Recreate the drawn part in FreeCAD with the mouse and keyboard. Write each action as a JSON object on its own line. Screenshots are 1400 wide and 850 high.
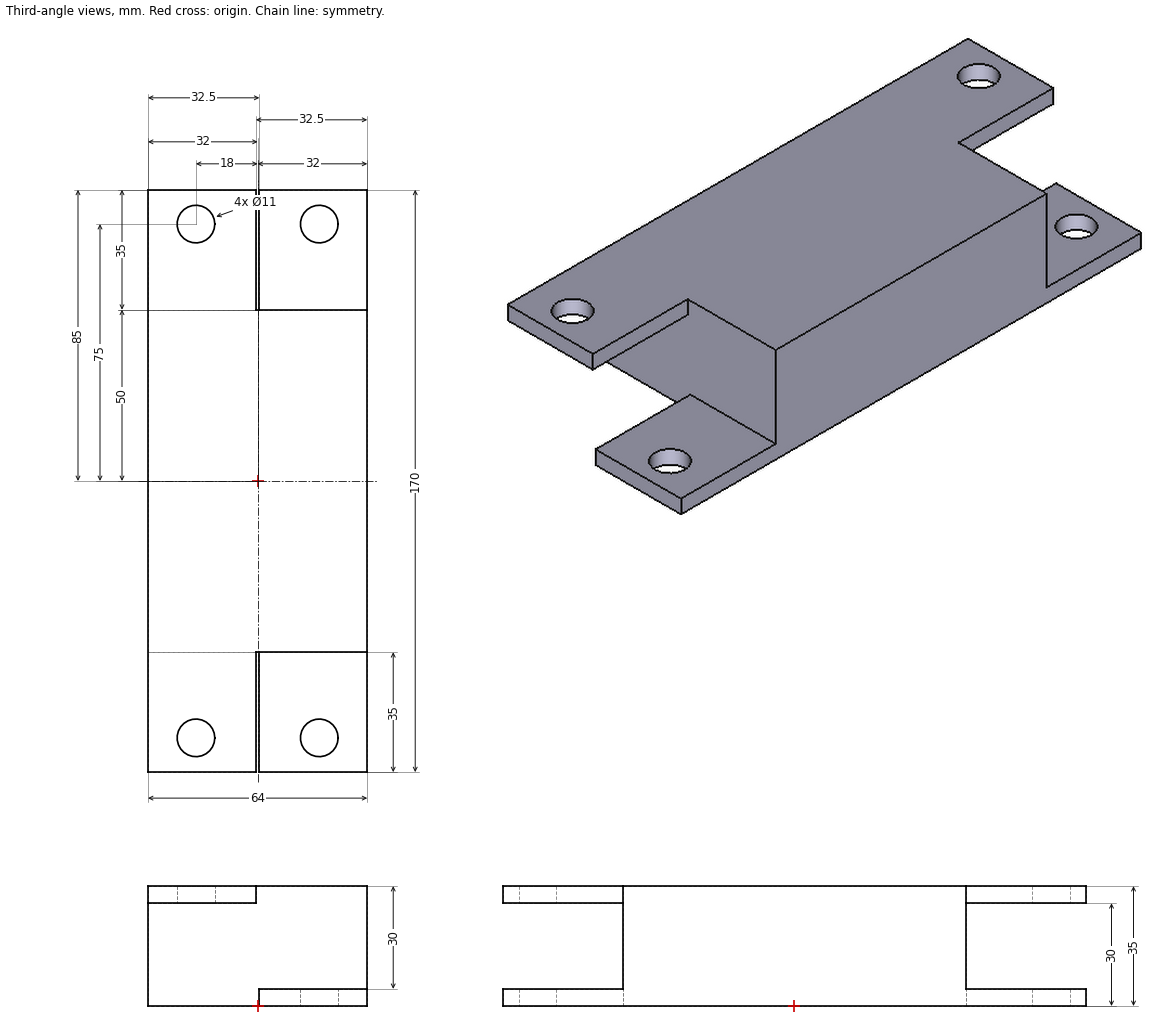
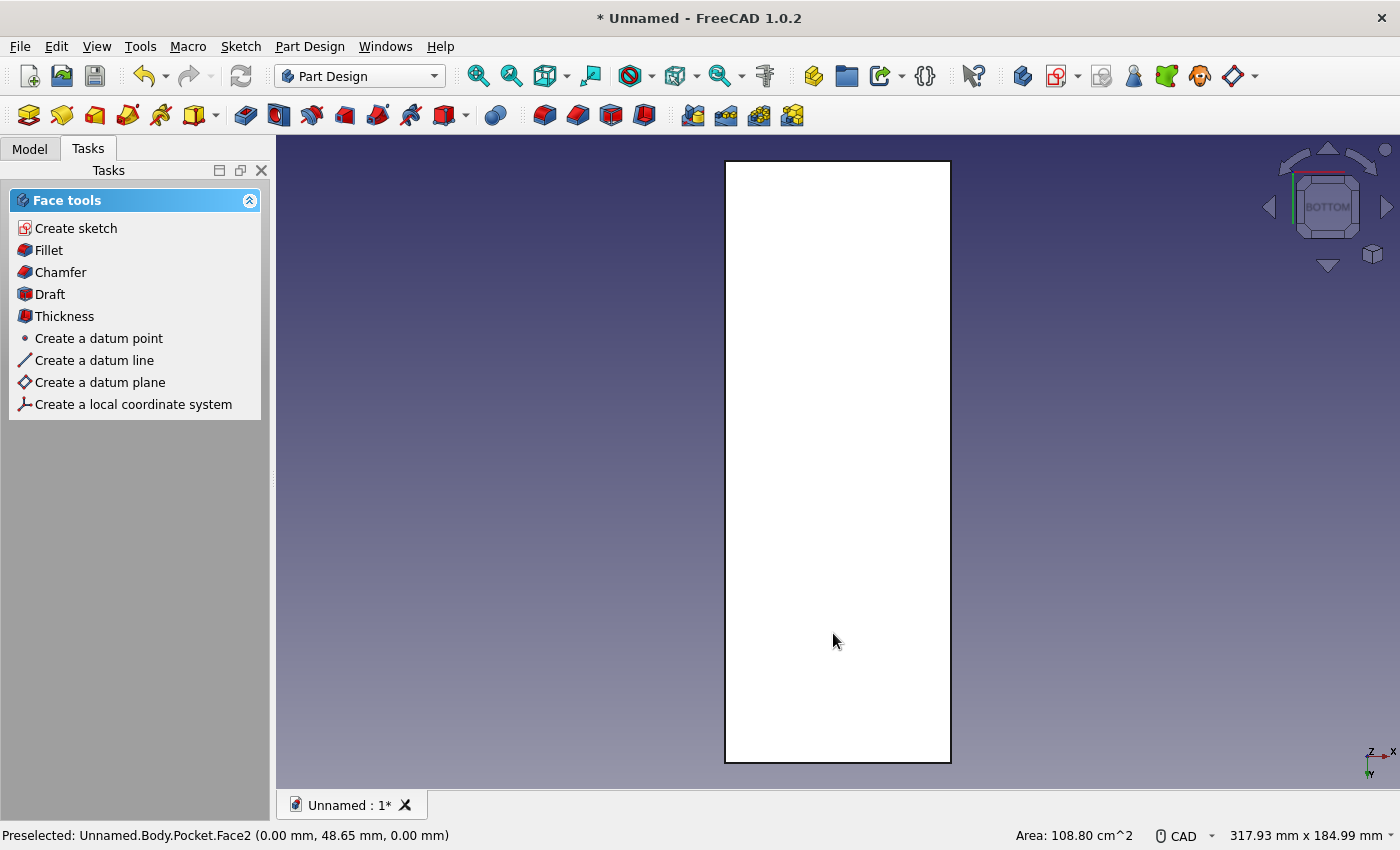
{"action": "left_click", "coordinate": [1056, 76]}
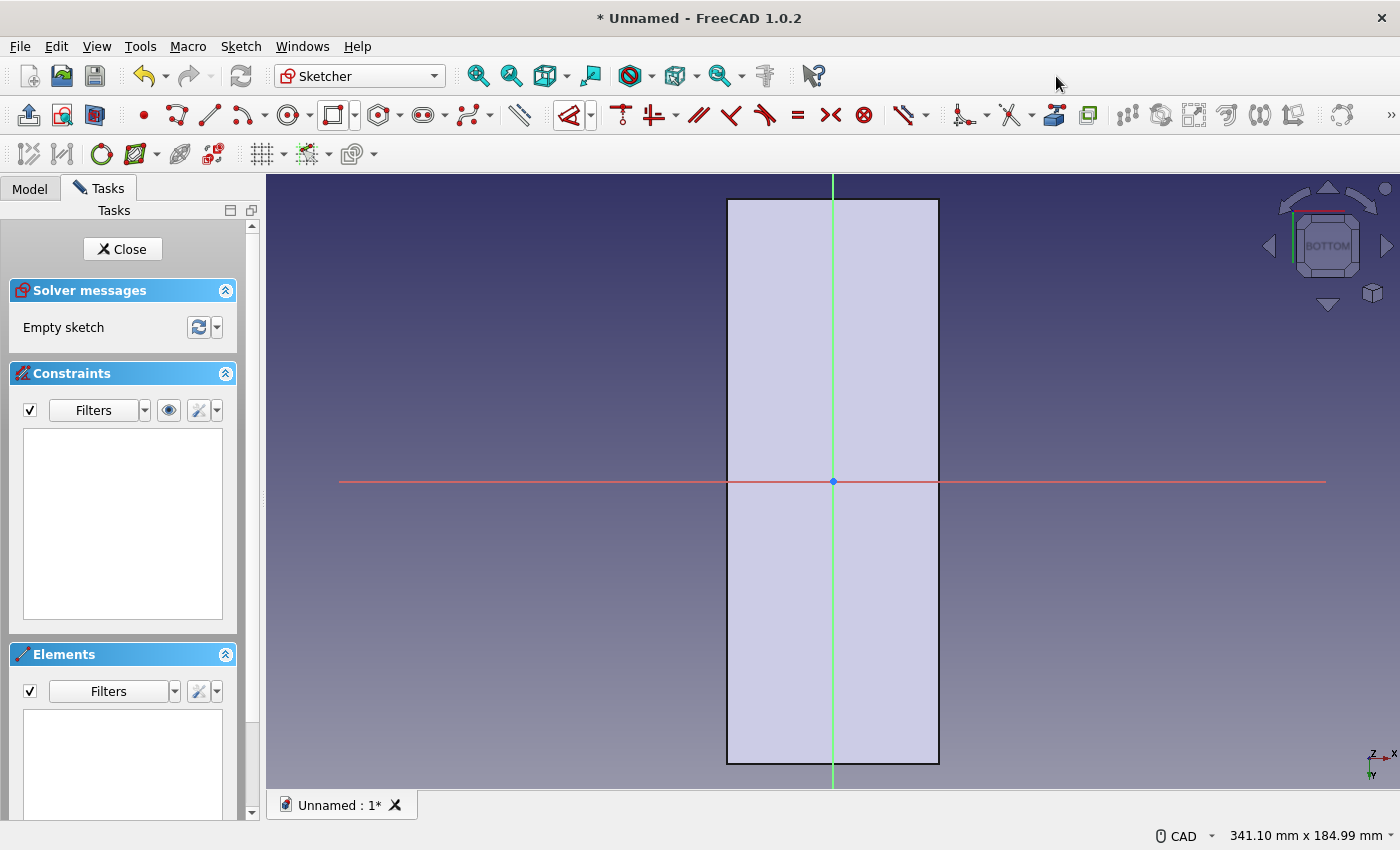
{"action": "scroll", "coordinate": [732, 481], "scroll_direction": "down", "scroll_amount": 2}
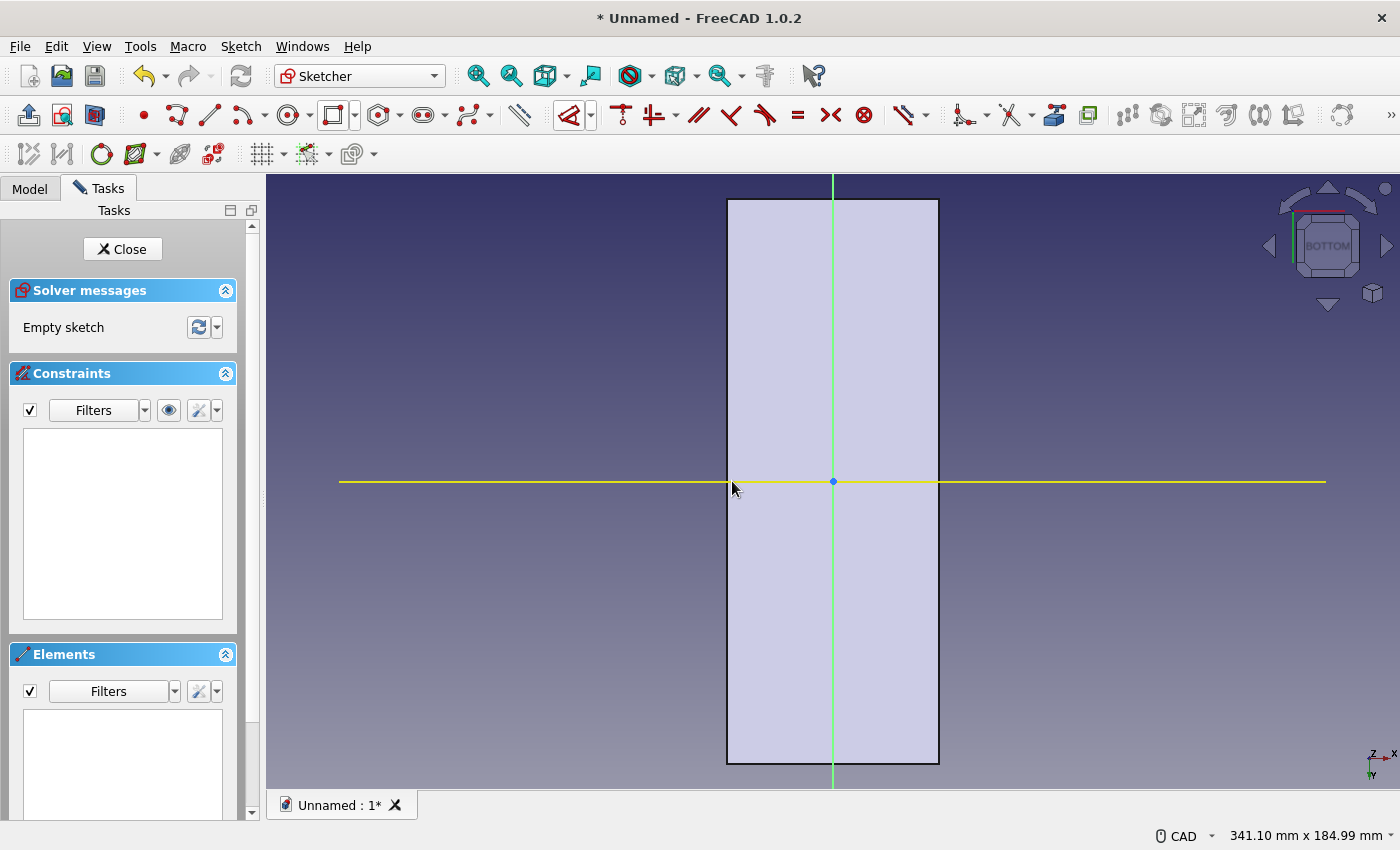
{"action": "left_click", "coordinate": [332, 116]}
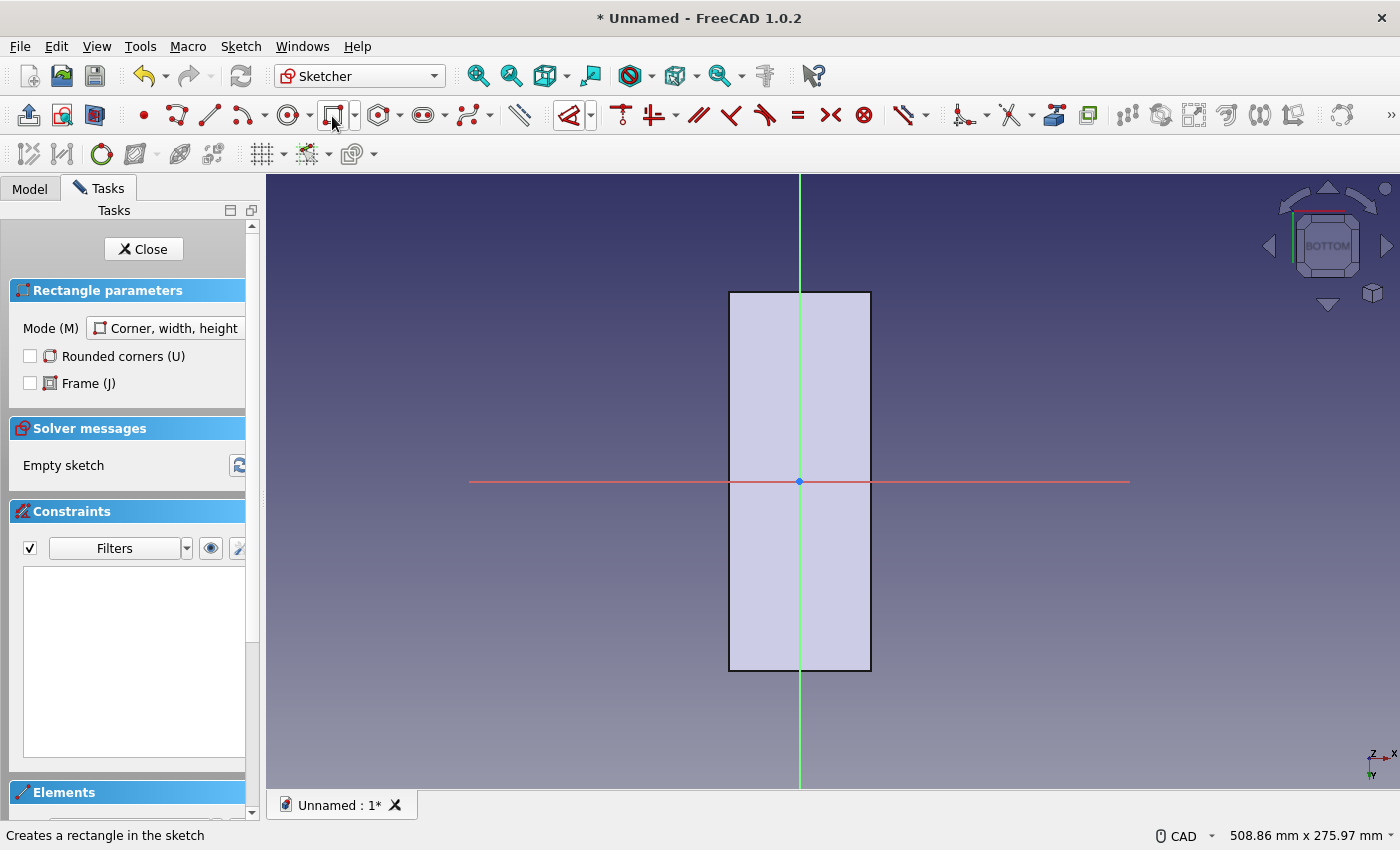
{"action": "left_click", "coordinate": [729, 593]}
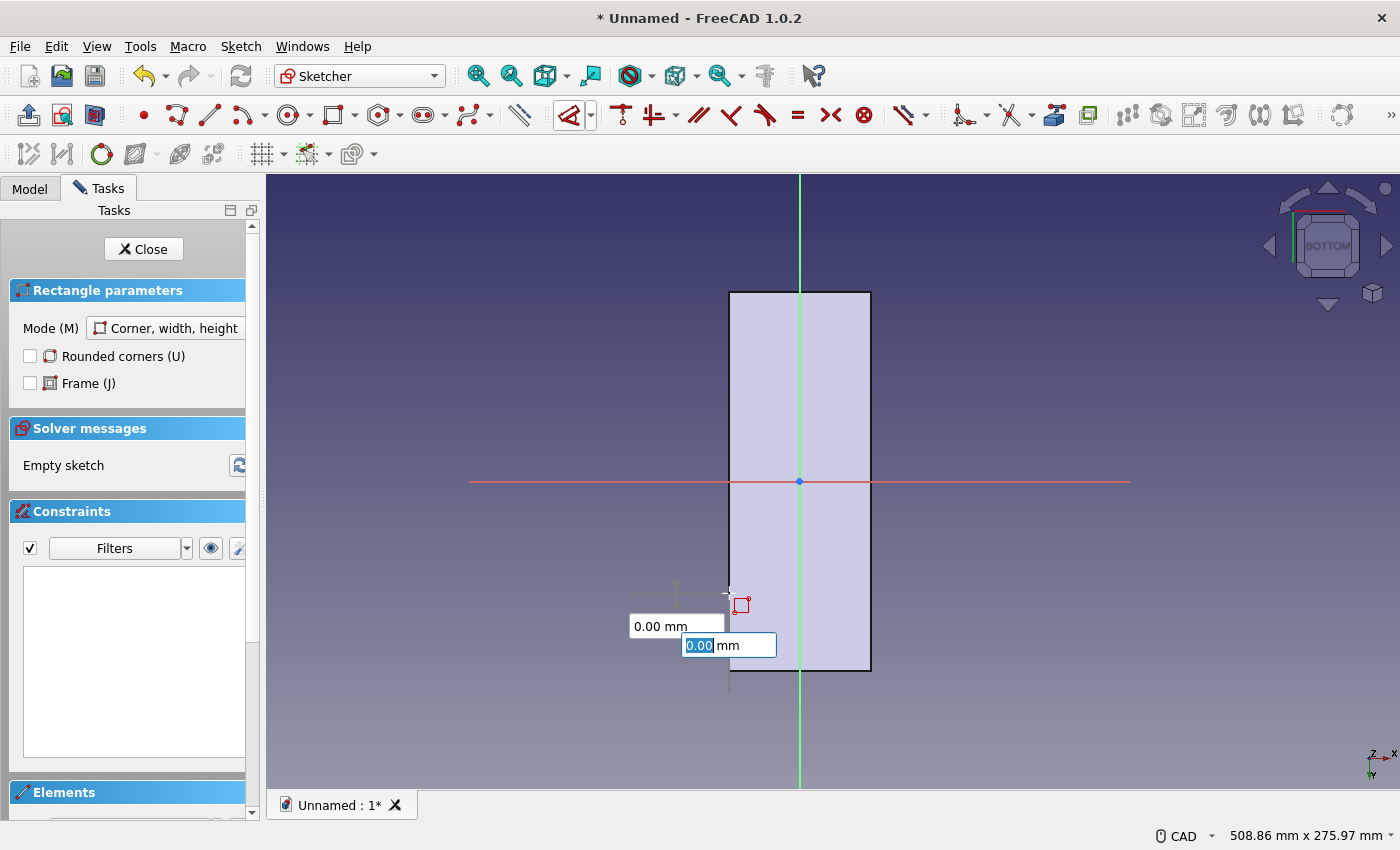
{"action": "scroll", "coordinate": [801, 671], "scroll_direction": "up", "scroll_amount": 14}
{"action": "mouse_move", "coordinate": [793, 657]}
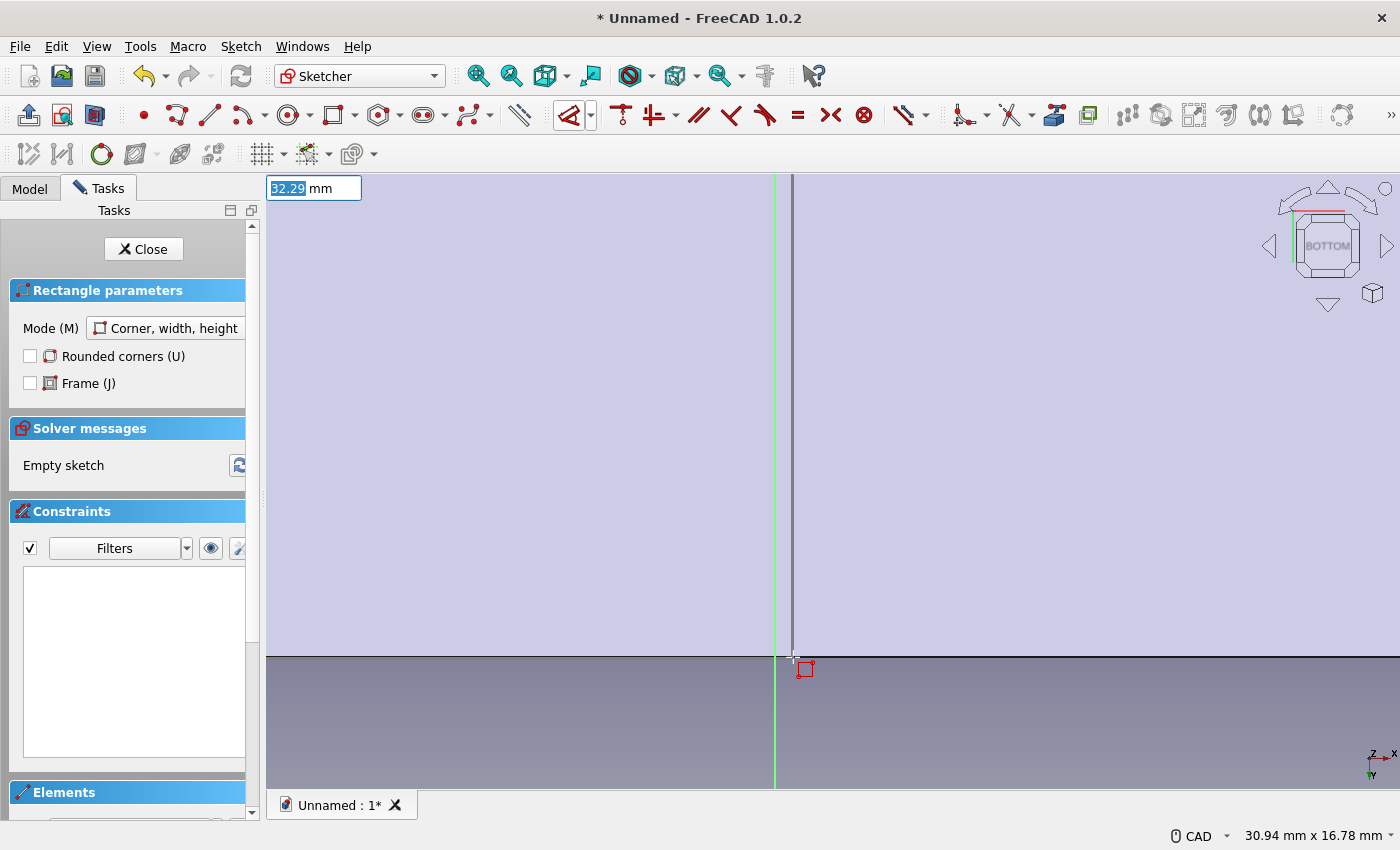
{"action": "type", "text": "32.5"}
{"action": "key", "text": "Tab"}
{"action": "type", "text": "35"}
{"action": "key", "text": "Return"}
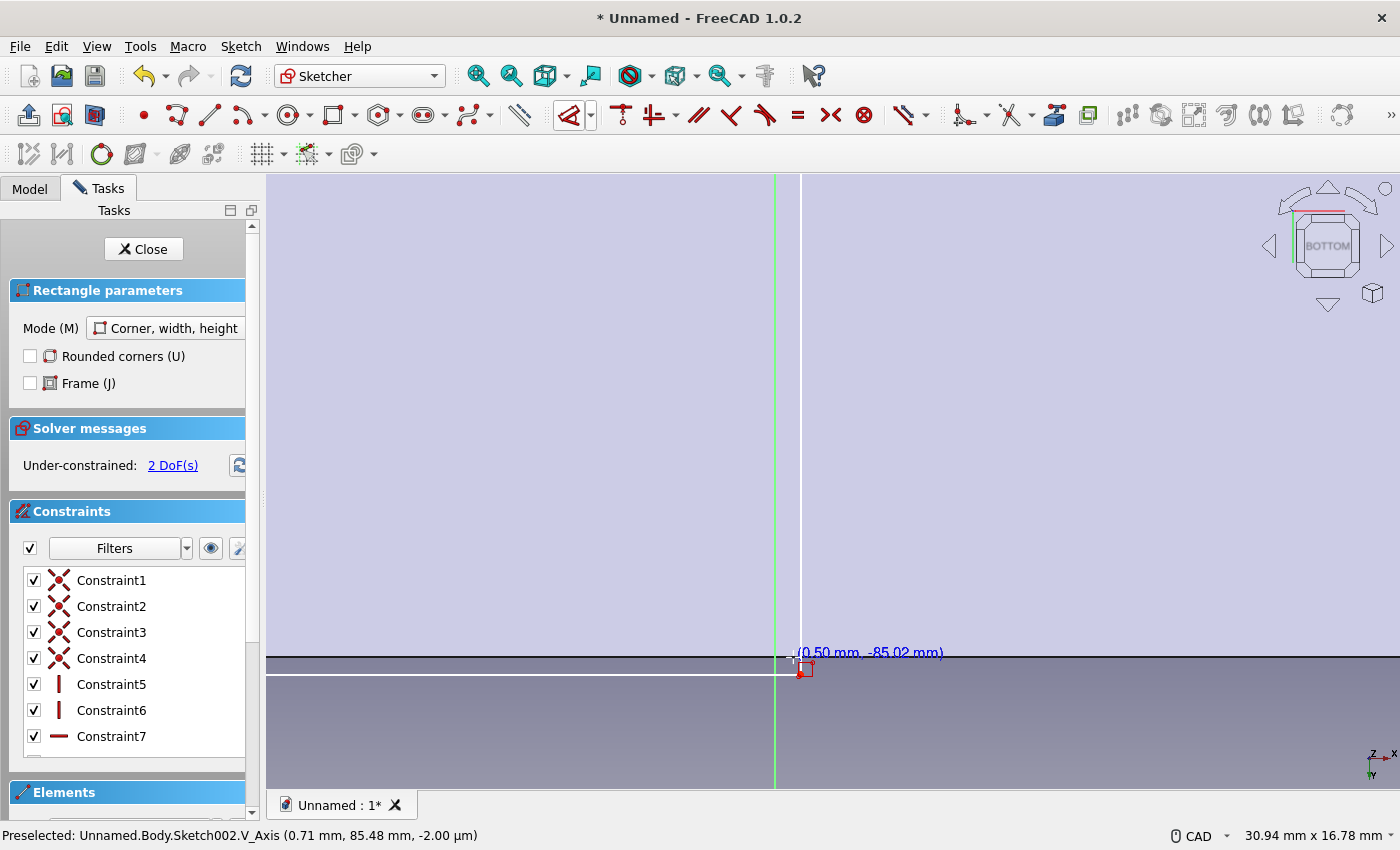
{"action": "scroll", "coordinate": [801, 672], "scroll_direction": "down", "scroll_amount": 14}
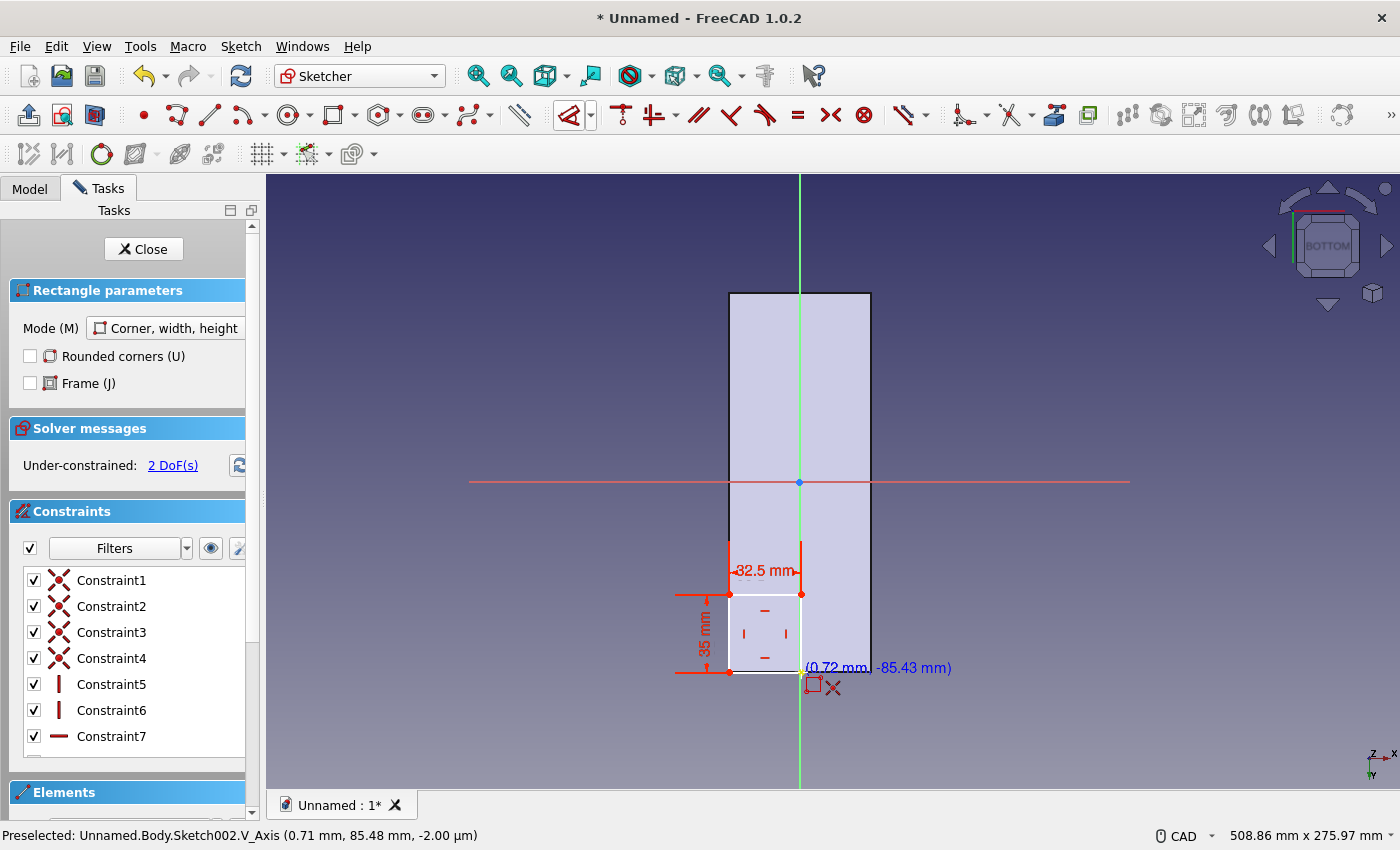
{"action": "left_click", "coordinate": [729, 293]}